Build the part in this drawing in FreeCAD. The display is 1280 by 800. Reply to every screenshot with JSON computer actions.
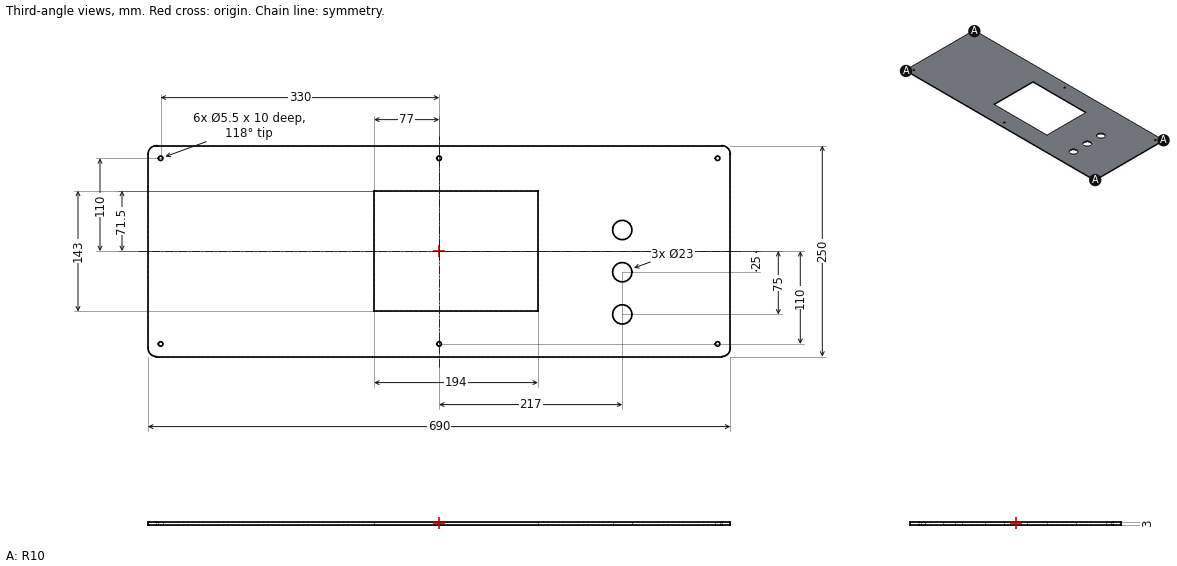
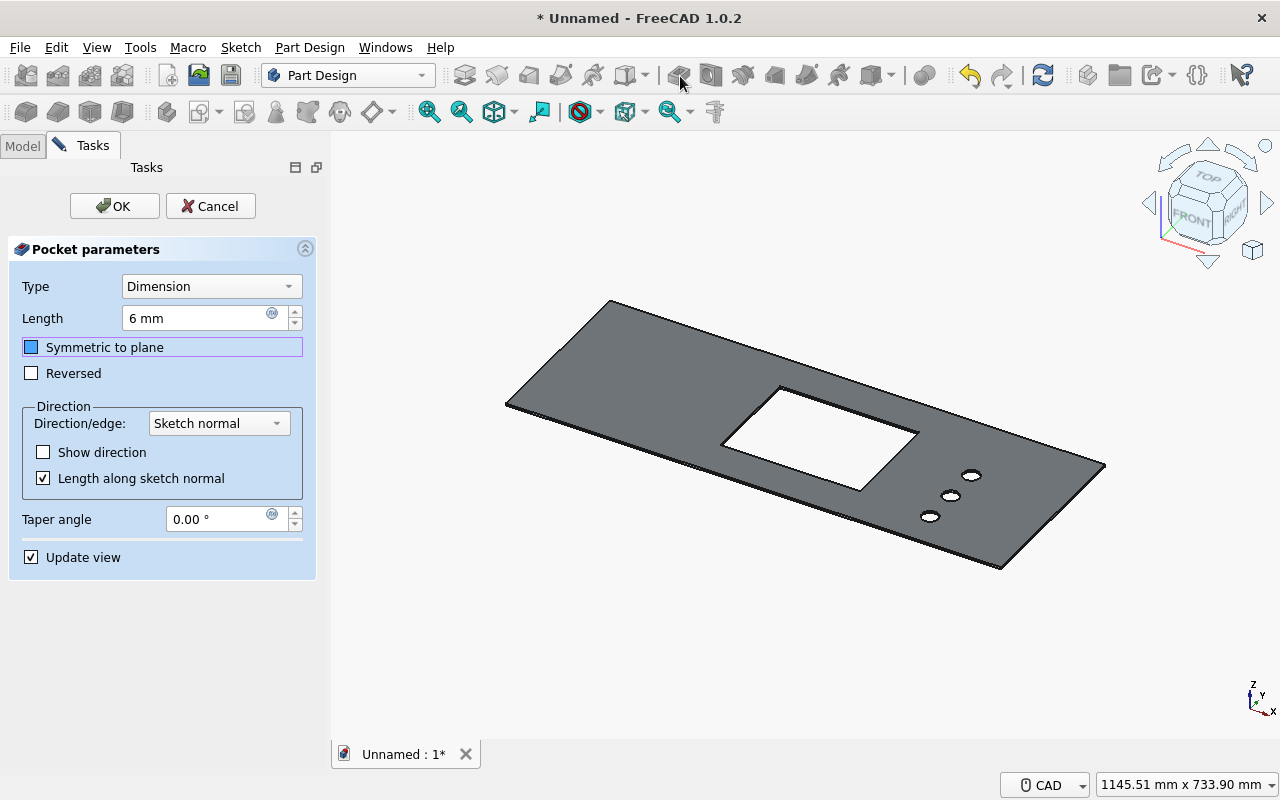
{"action": "left_click", "coordinate": [115, 206]}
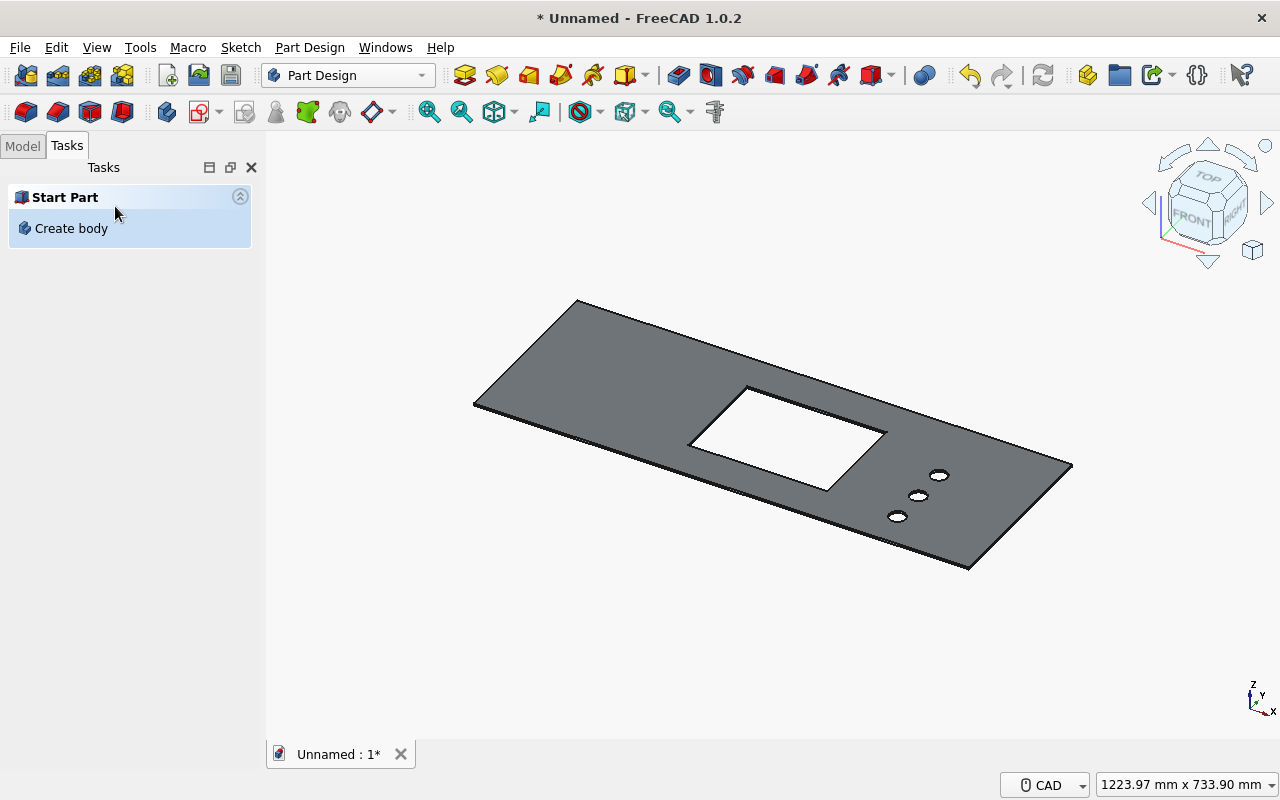
{"action": "scroll", "coordinate": [969, 567], "scroll_direction": "up", "scroll_amount": 14}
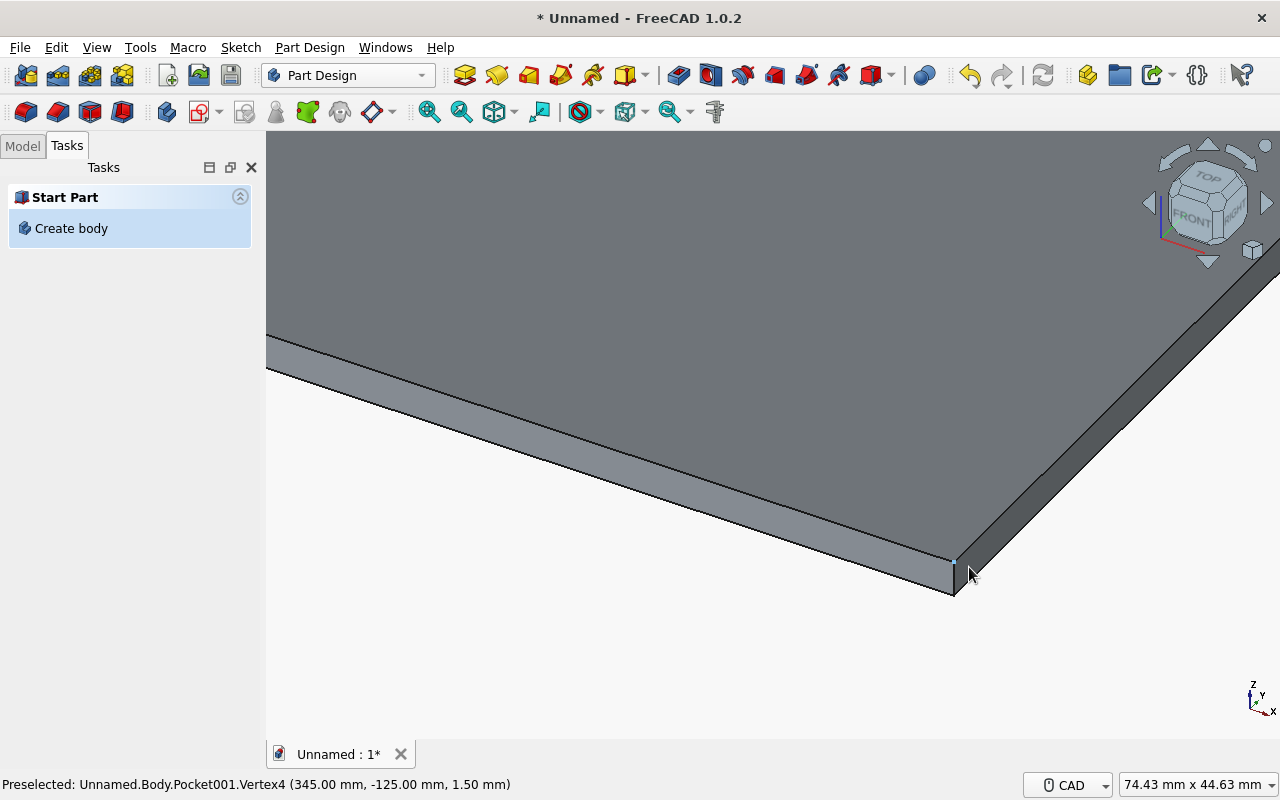
{"action": "left_click", "coordinate": [954, 578]}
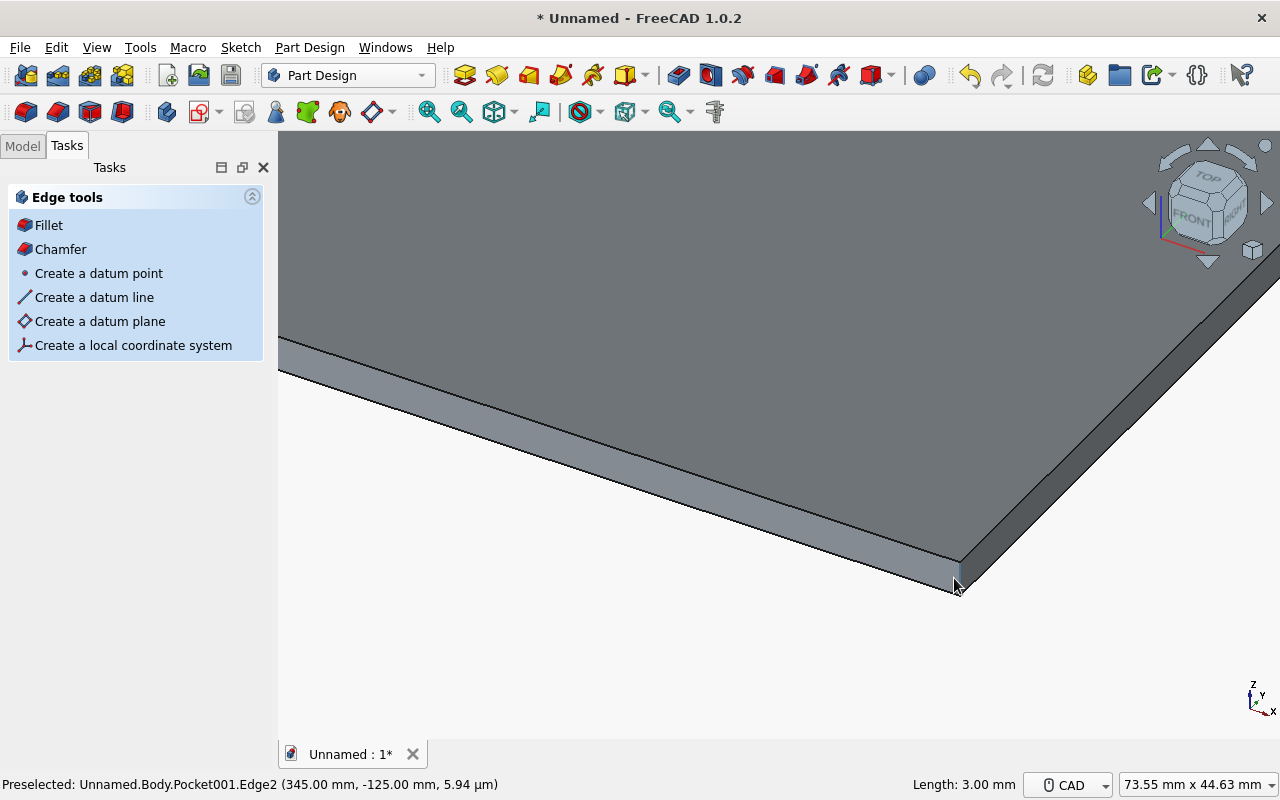
{"action": "left_click", "coordinate": [430, 112]}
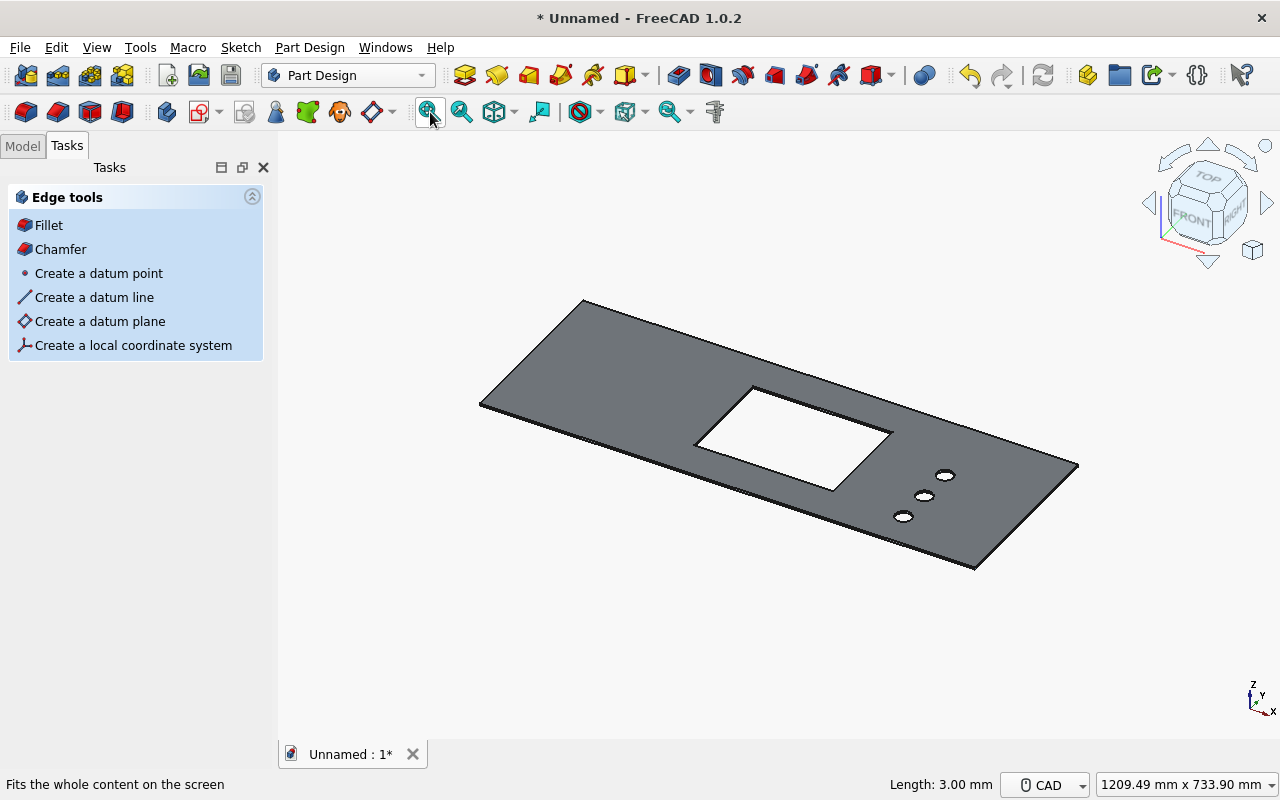
{"action": "key", "text": "0"}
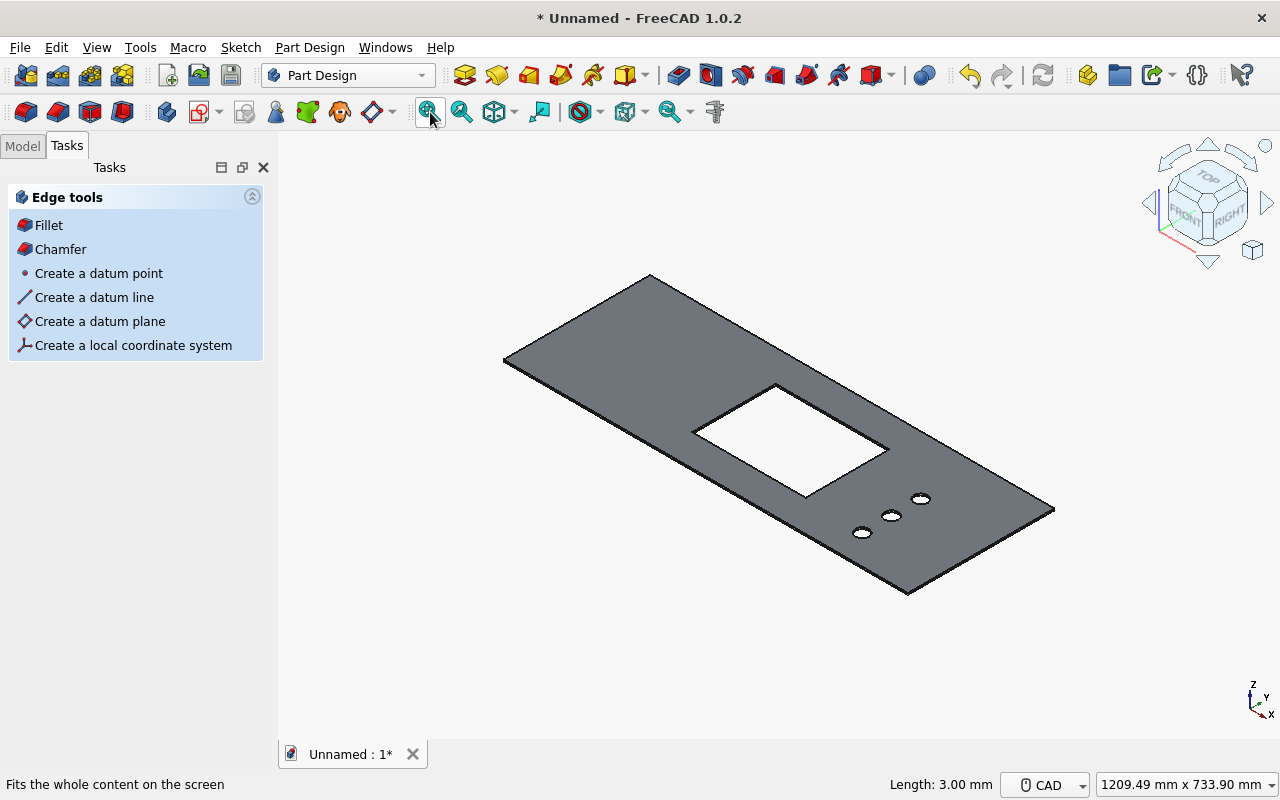
{"action": "scroll", "coordinate": [504, 360], "scroll_direction": "up", "scroll_amount": 14}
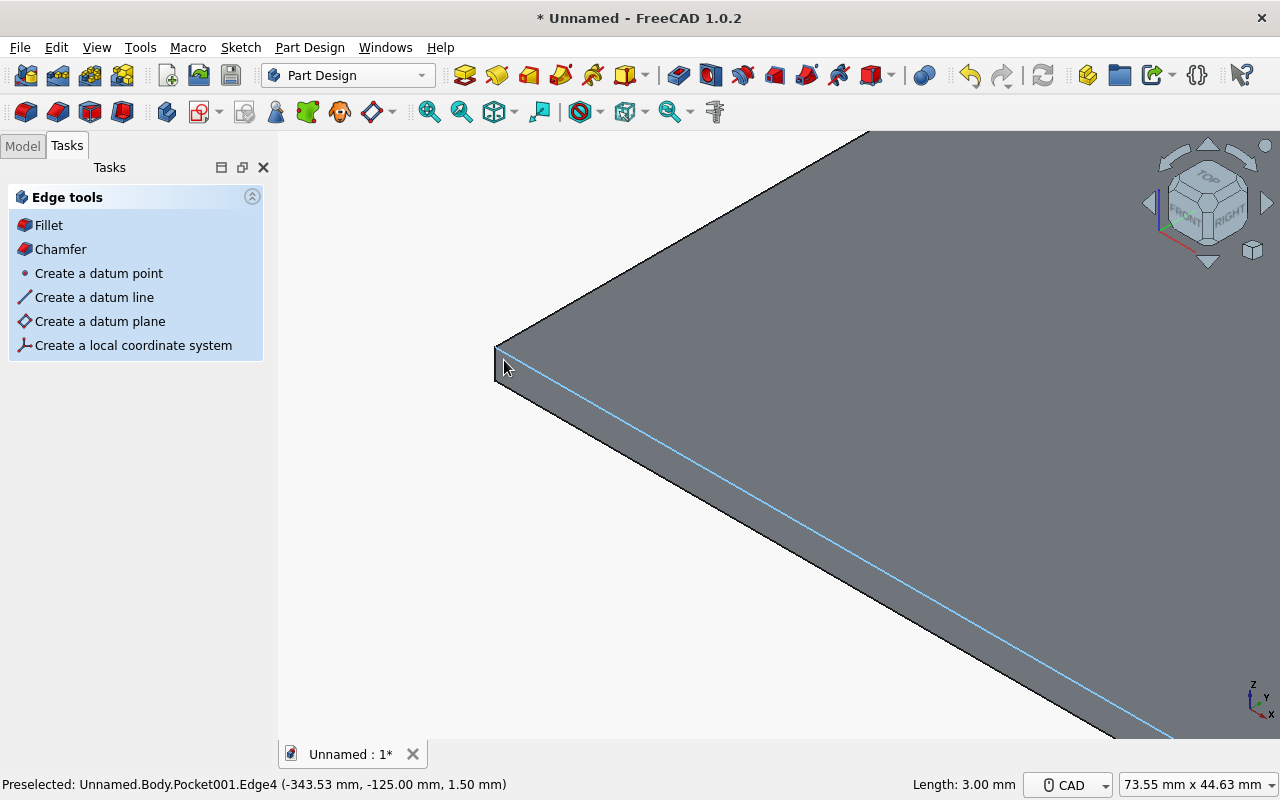
{"action": "left_click", "coordinate": [430, 112]}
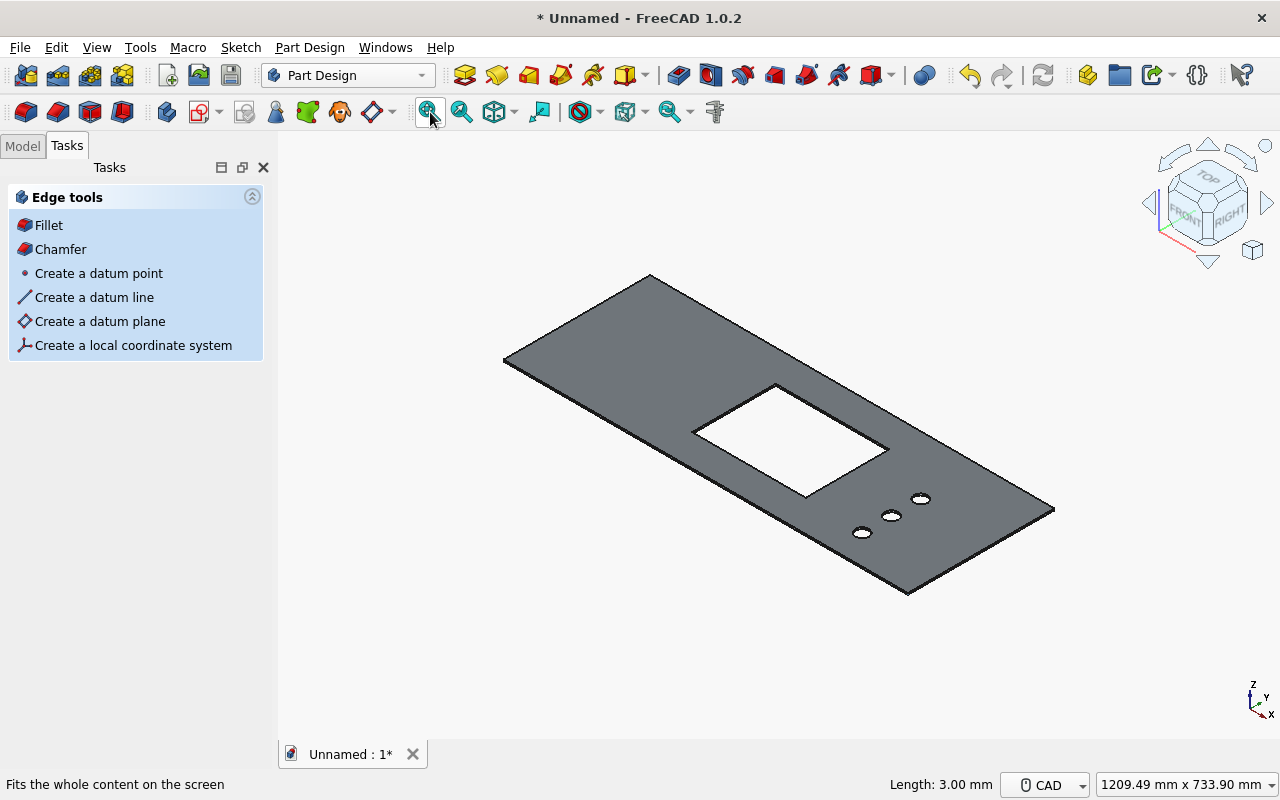
{"action": "key", "text": "2"}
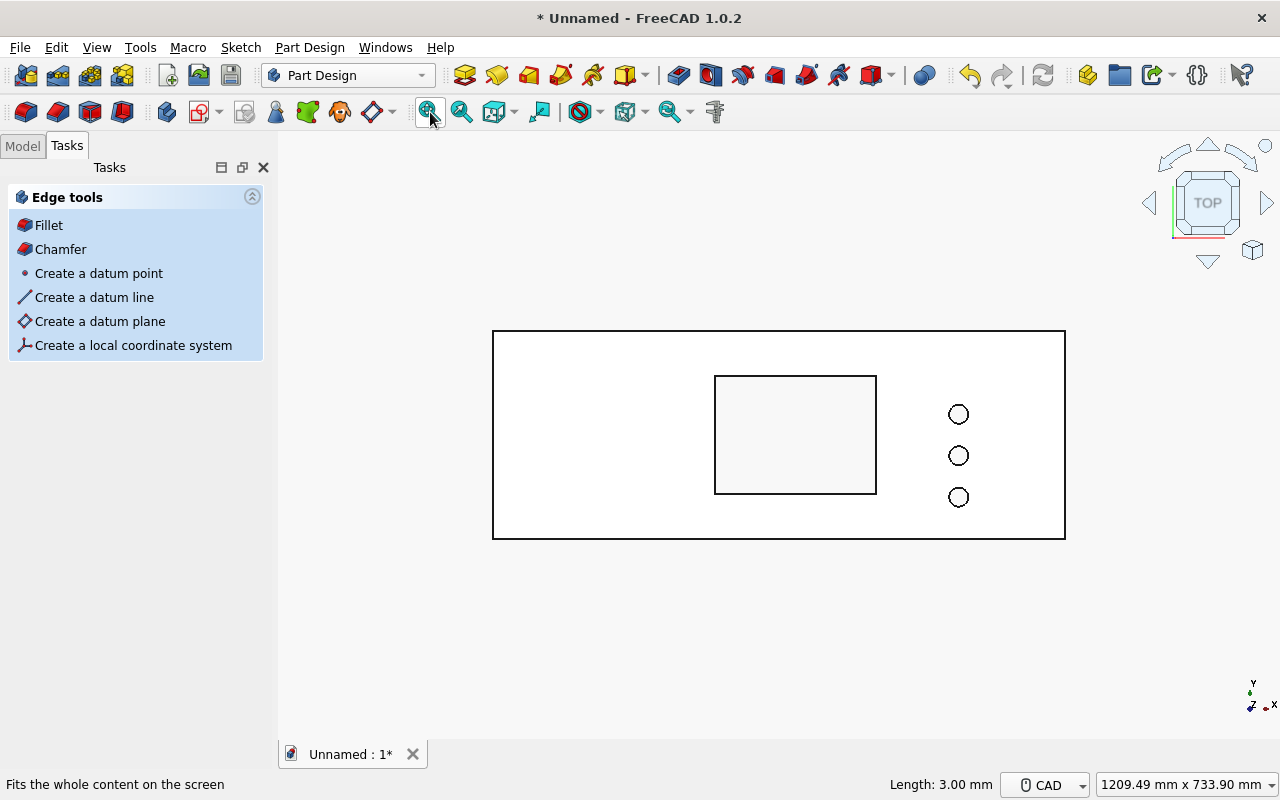
{"action": "scroll", "coordinate": [493, 538], "scroll_direction": "up", "scroll_amount": 14}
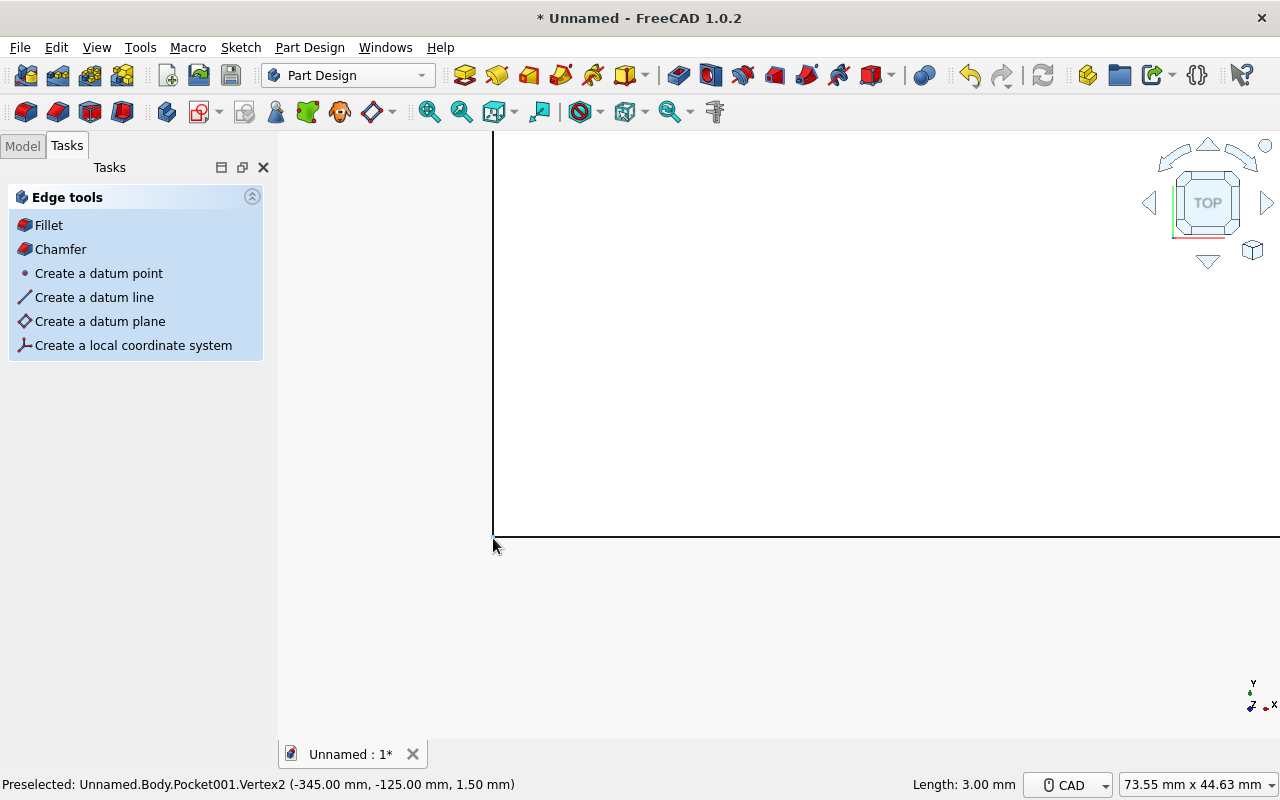
{"action": "left_click", "coordinate": [430, 112]}